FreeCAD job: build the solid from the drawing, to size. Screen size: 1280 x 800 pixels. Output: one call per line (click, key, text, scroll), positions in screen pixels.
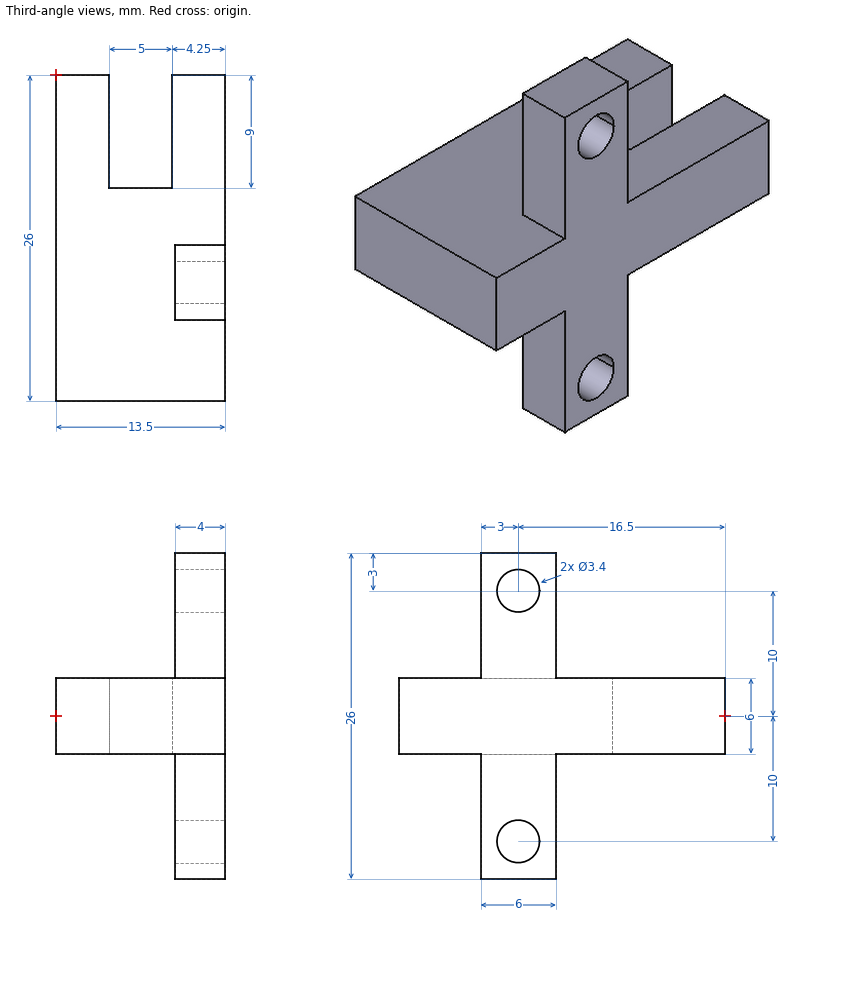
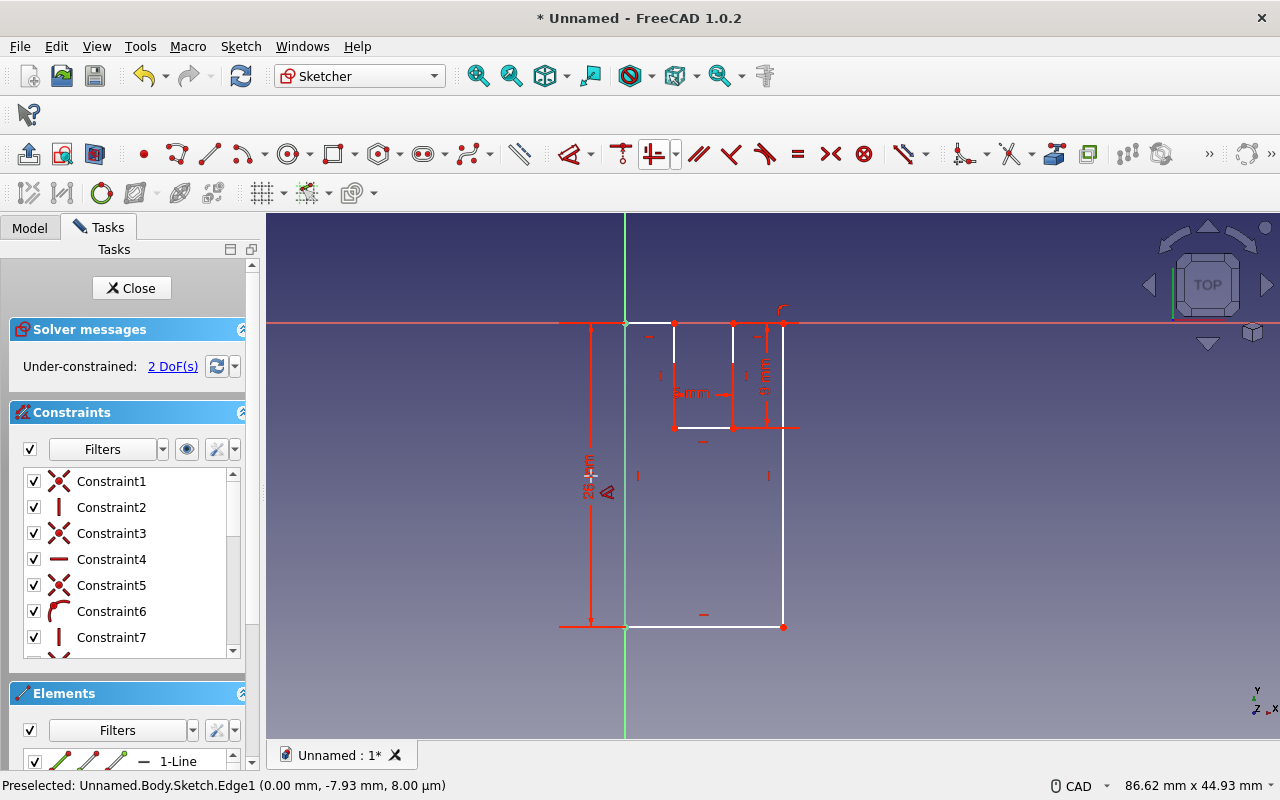
click(673, 627)
click(704, 661)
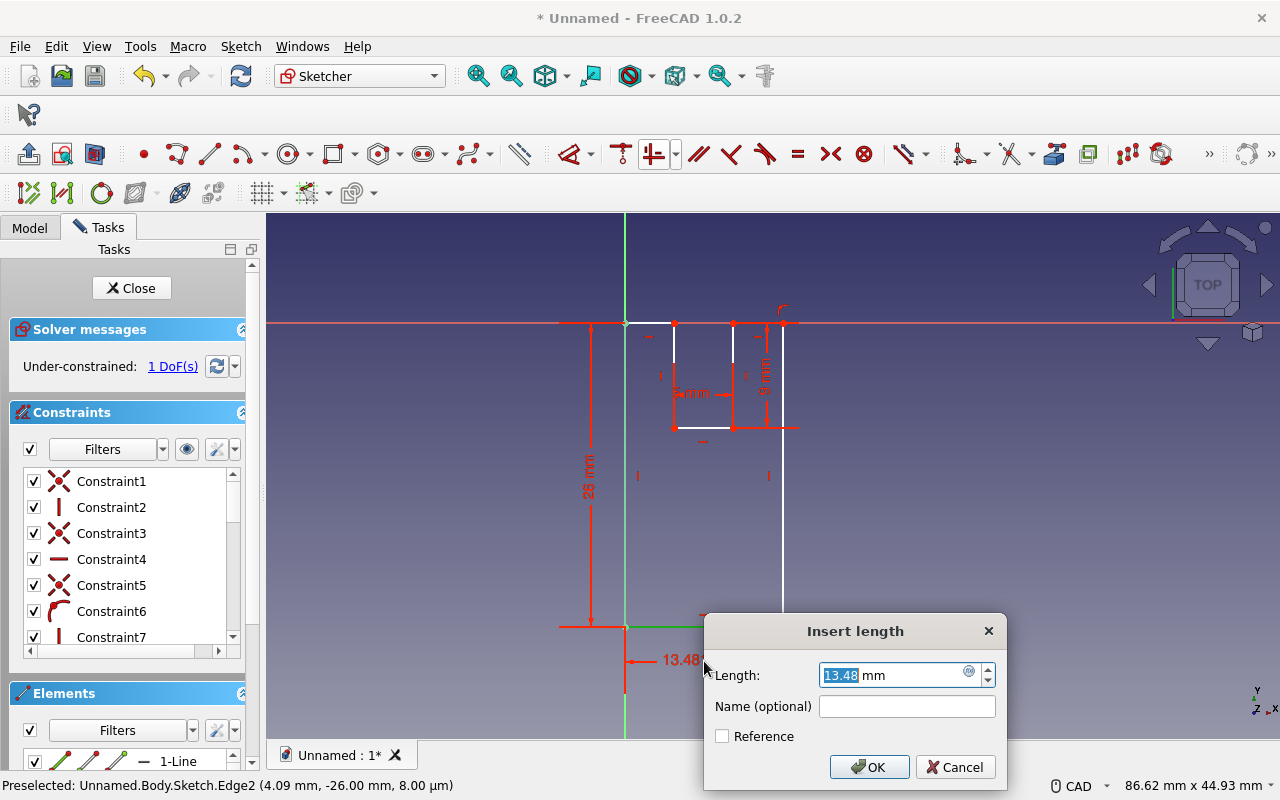
text(13.5)
key(Return)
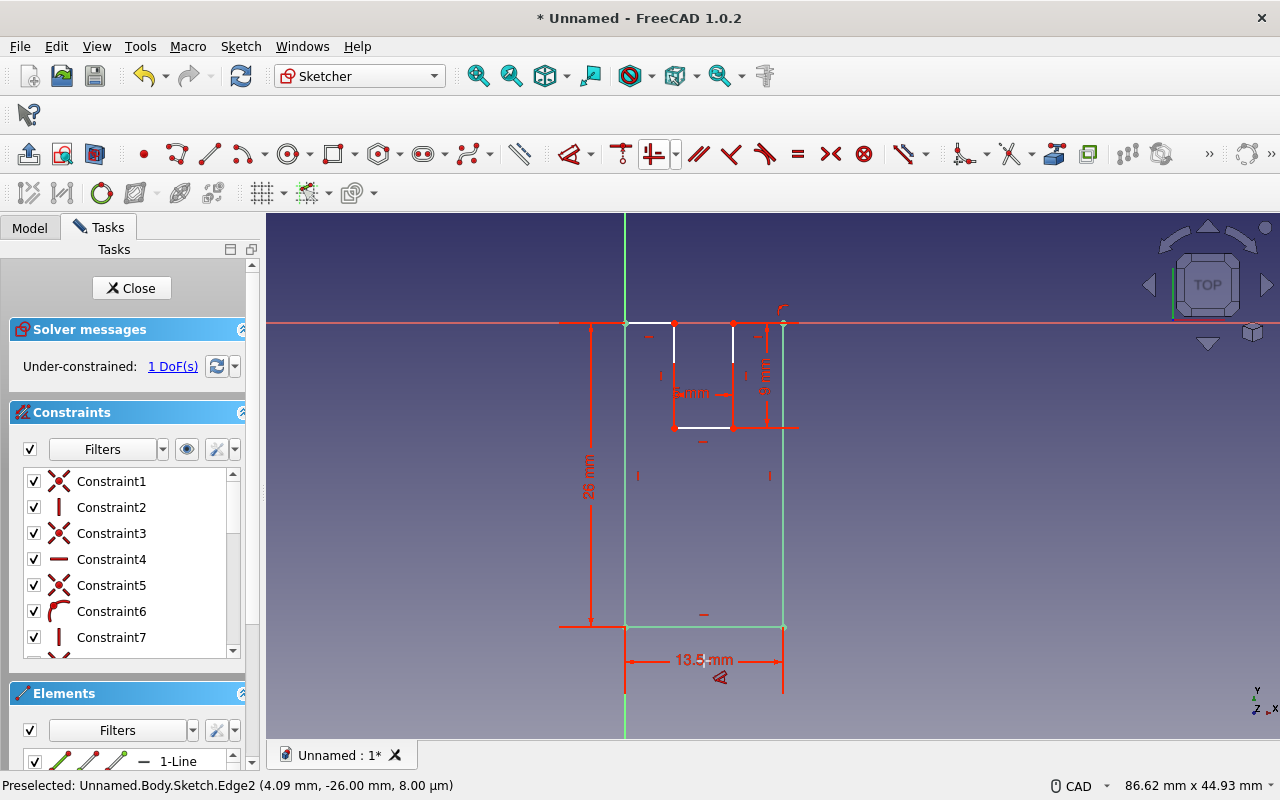
click(768, 323)
click(758, 289)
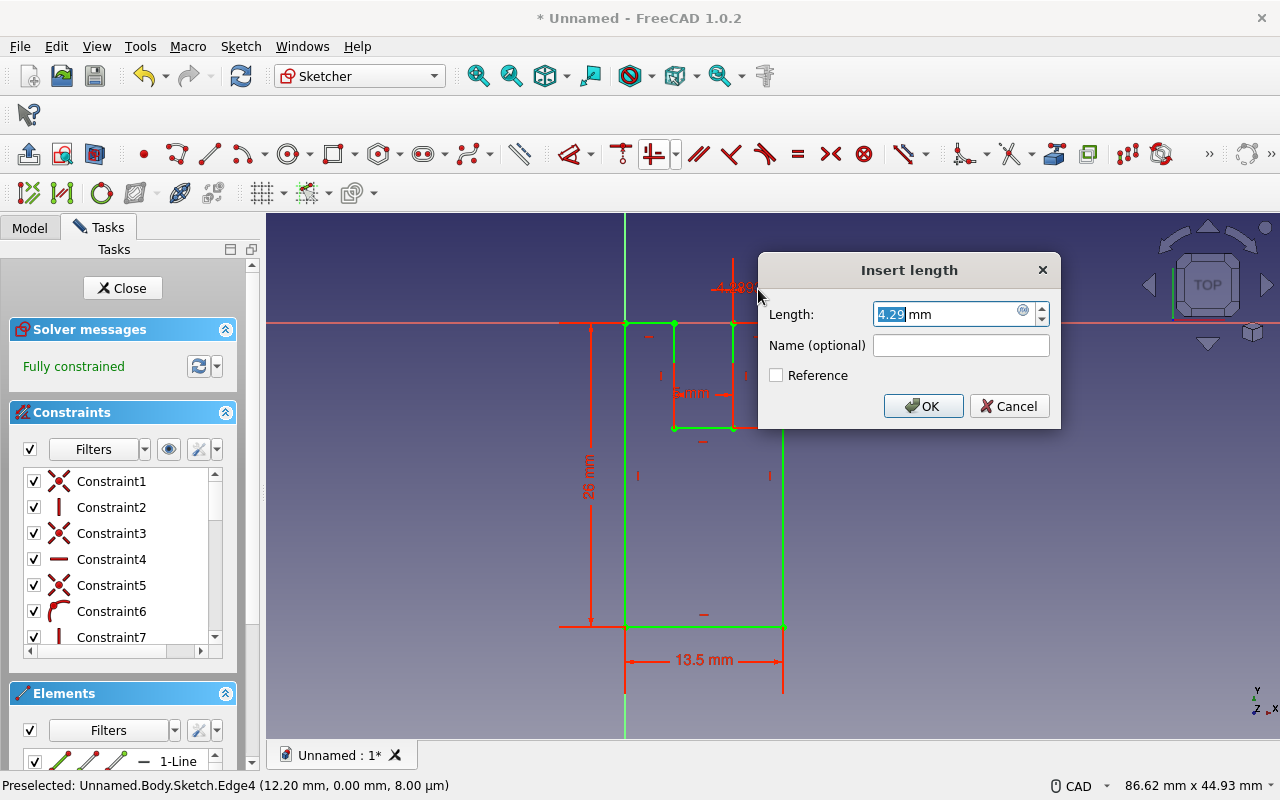
text(4.25)
key(Return)
key(Escape)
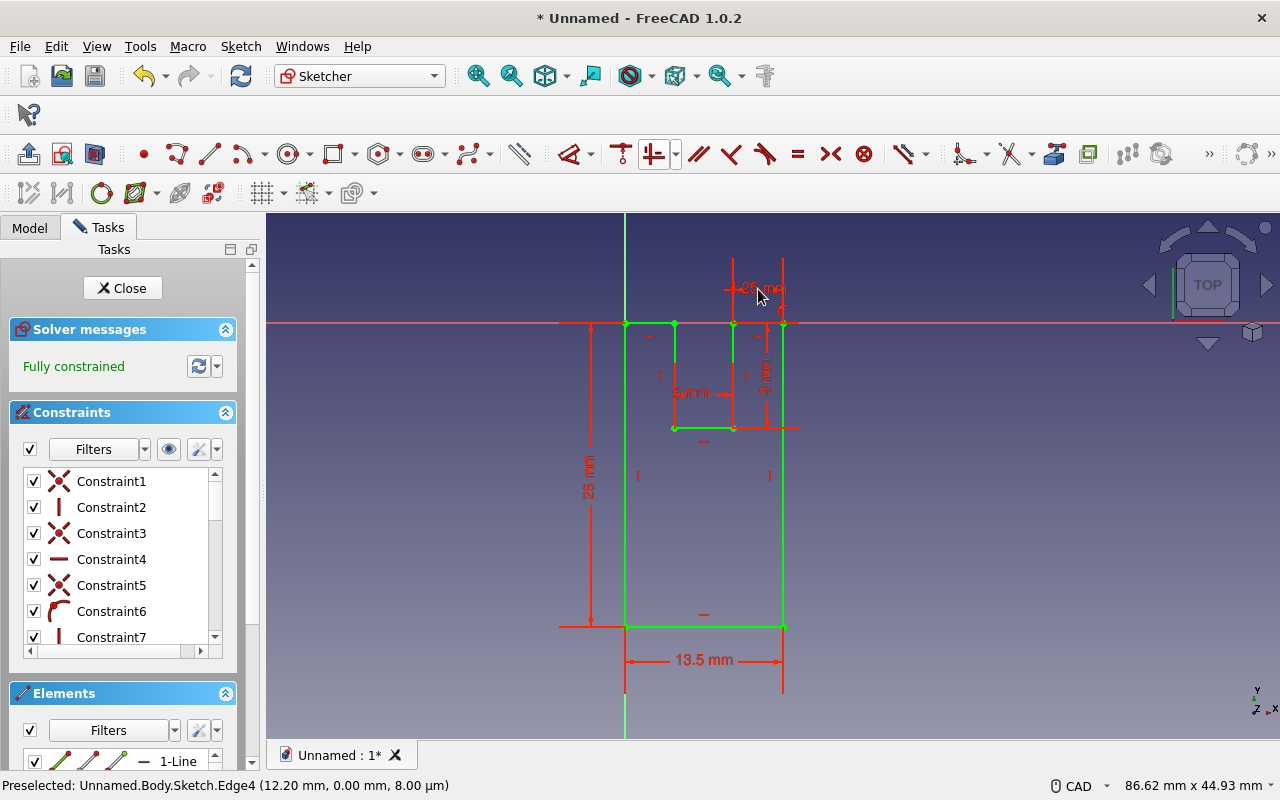
click(123, 288)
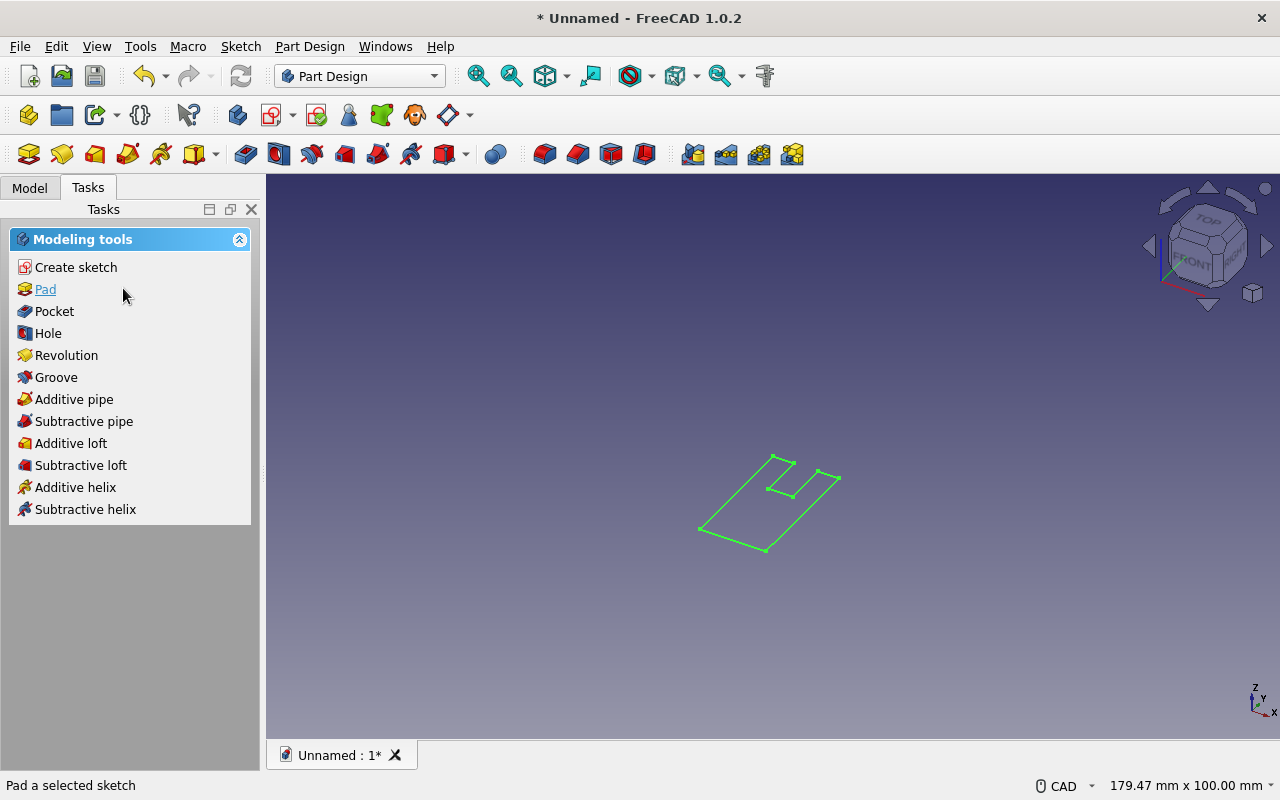
click(29, 154)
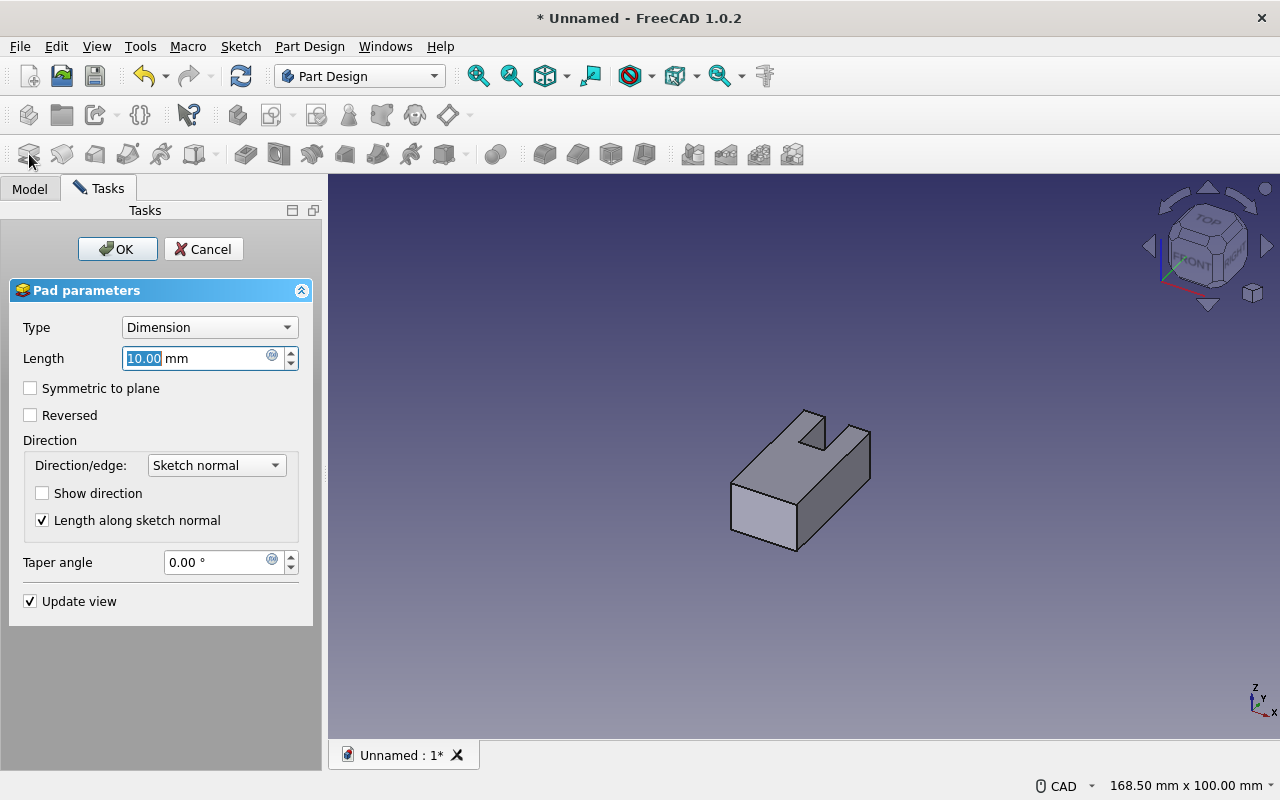
text(6)
key(Tab)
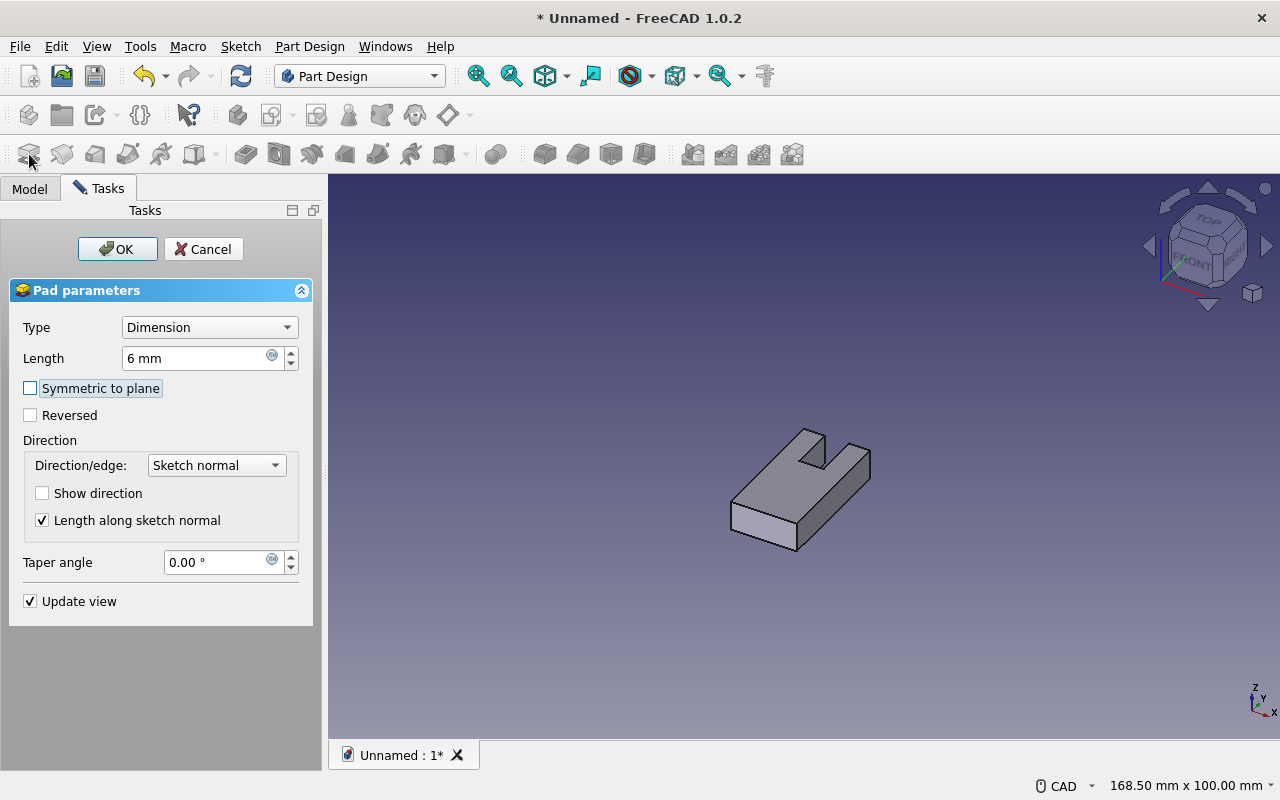
click(31, 388)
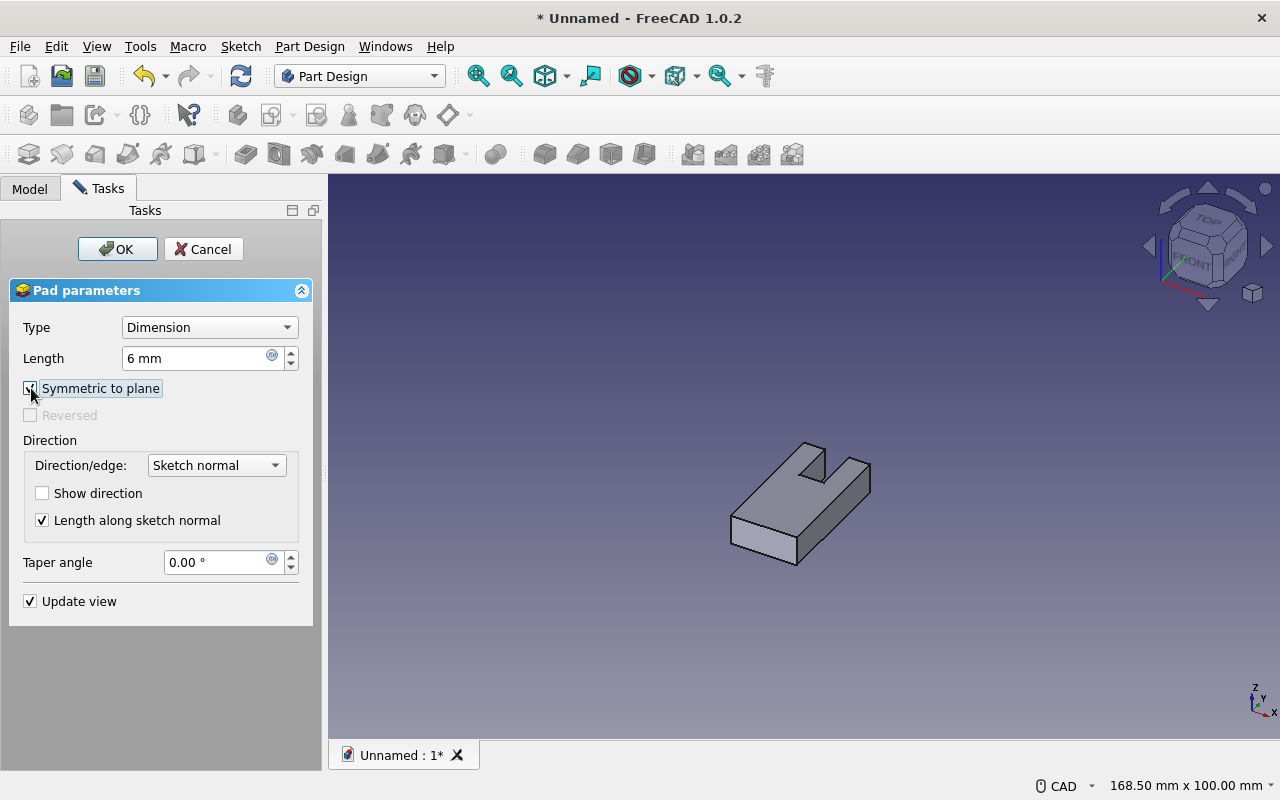
click(118, 249)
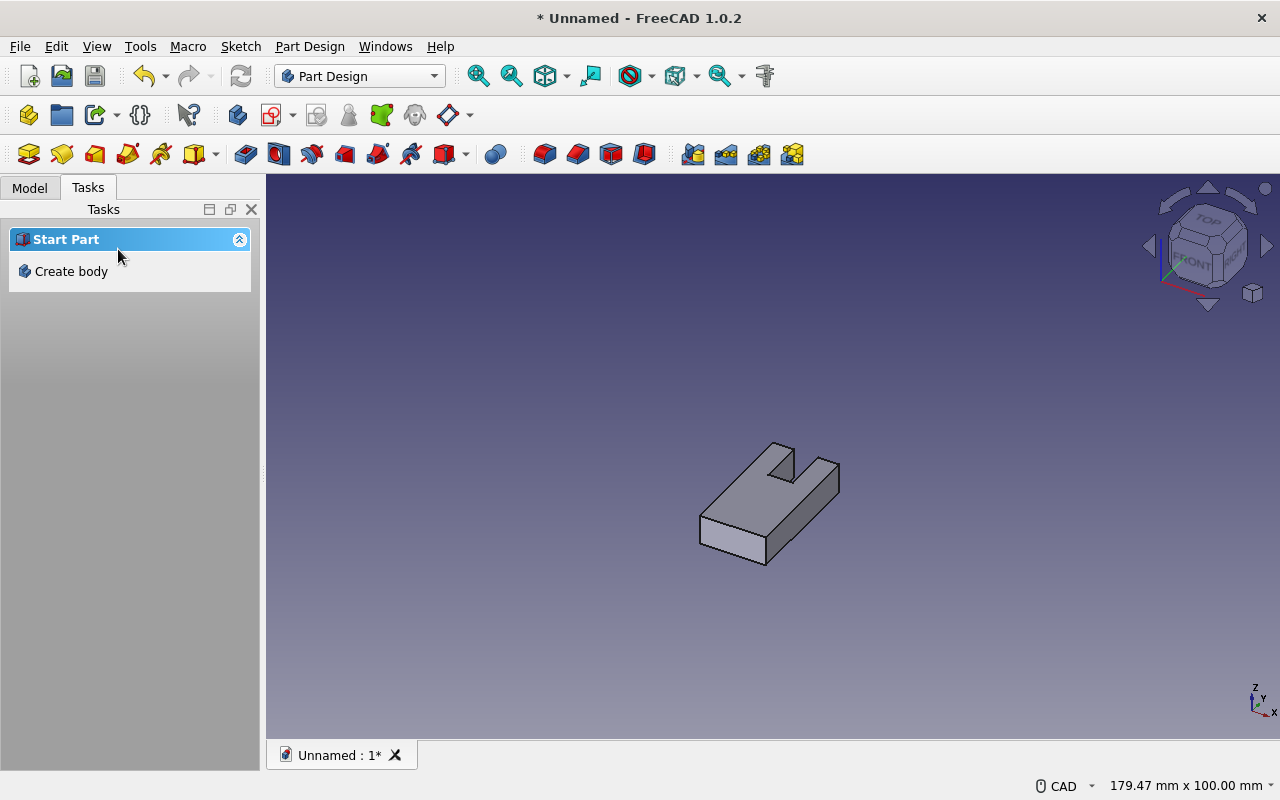
click(479, 76)